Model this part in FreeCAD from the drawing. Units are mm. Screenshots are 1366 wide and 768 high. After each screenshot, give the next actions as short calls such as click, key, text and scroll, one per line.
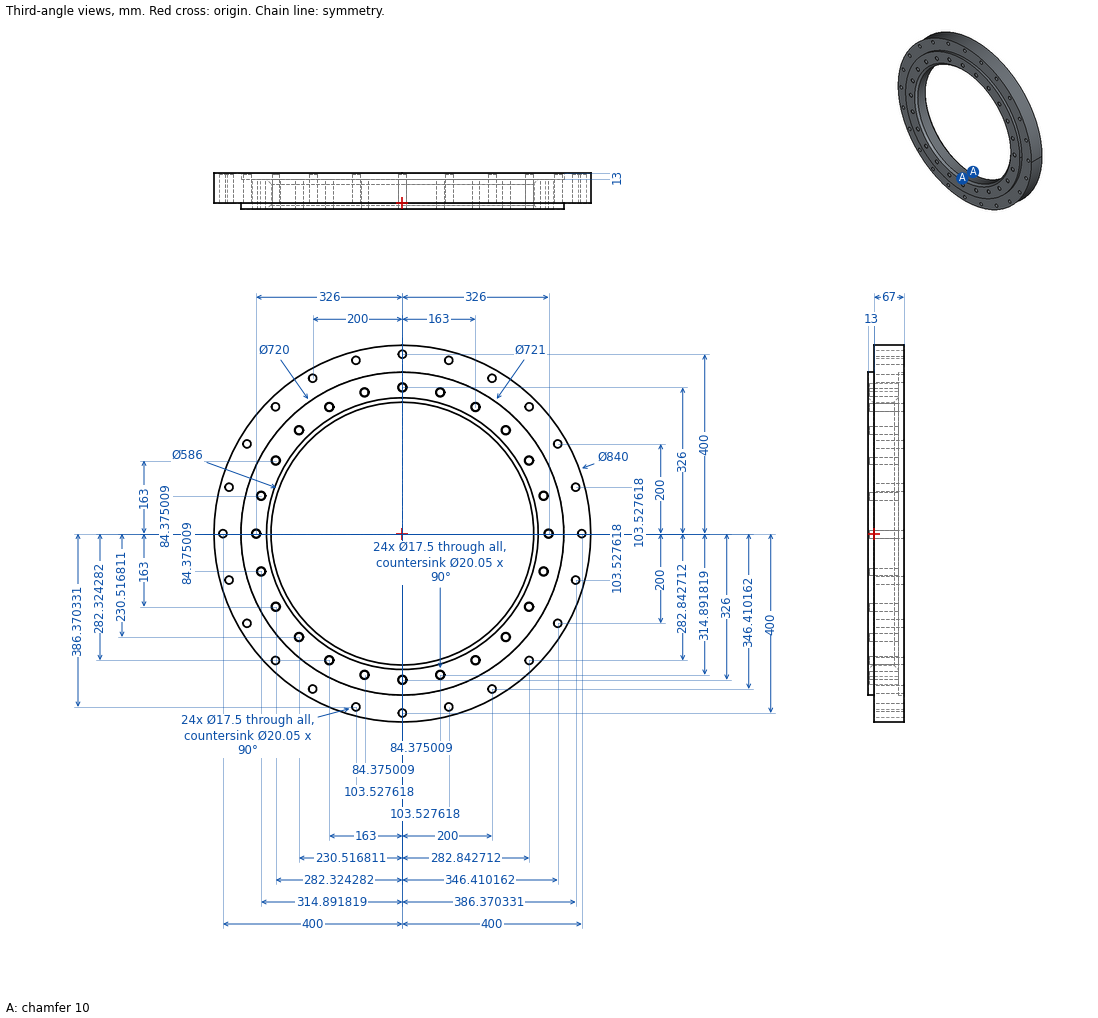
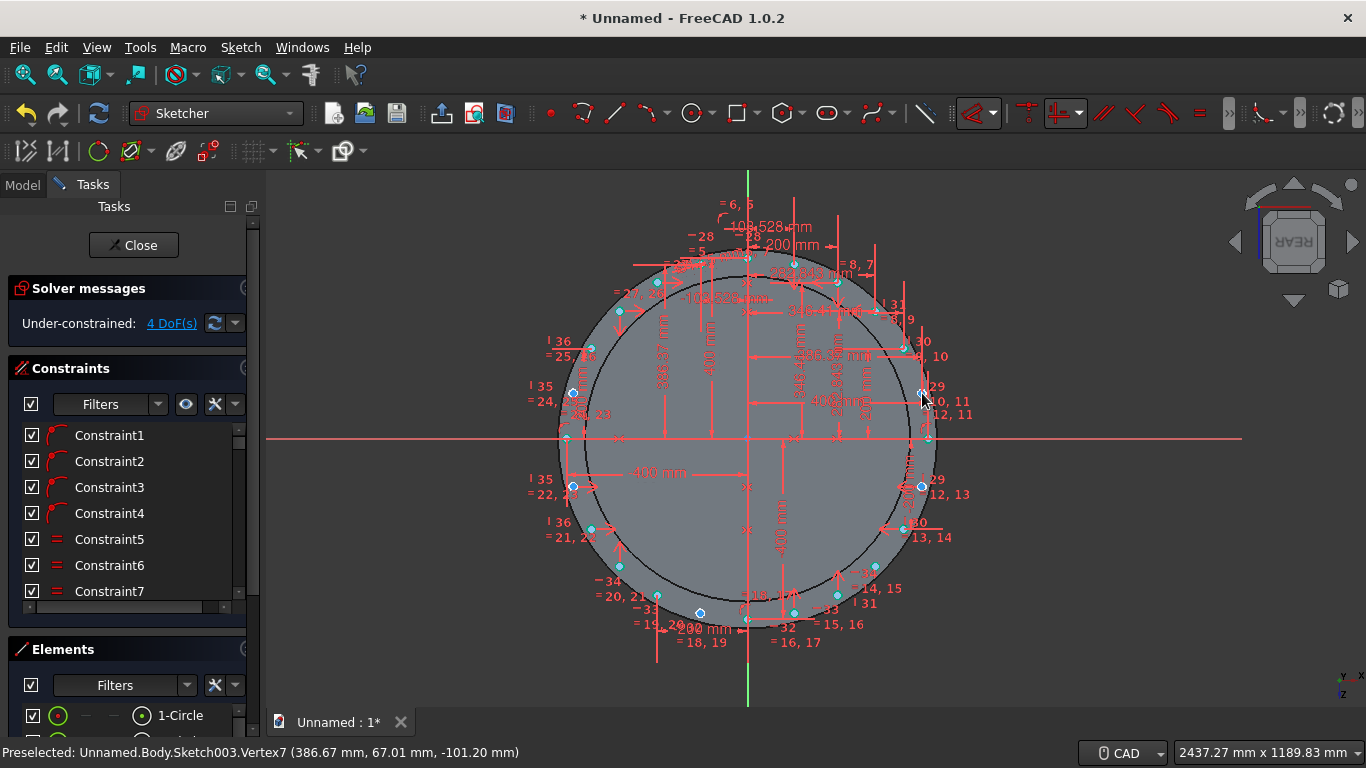
click(922, 393)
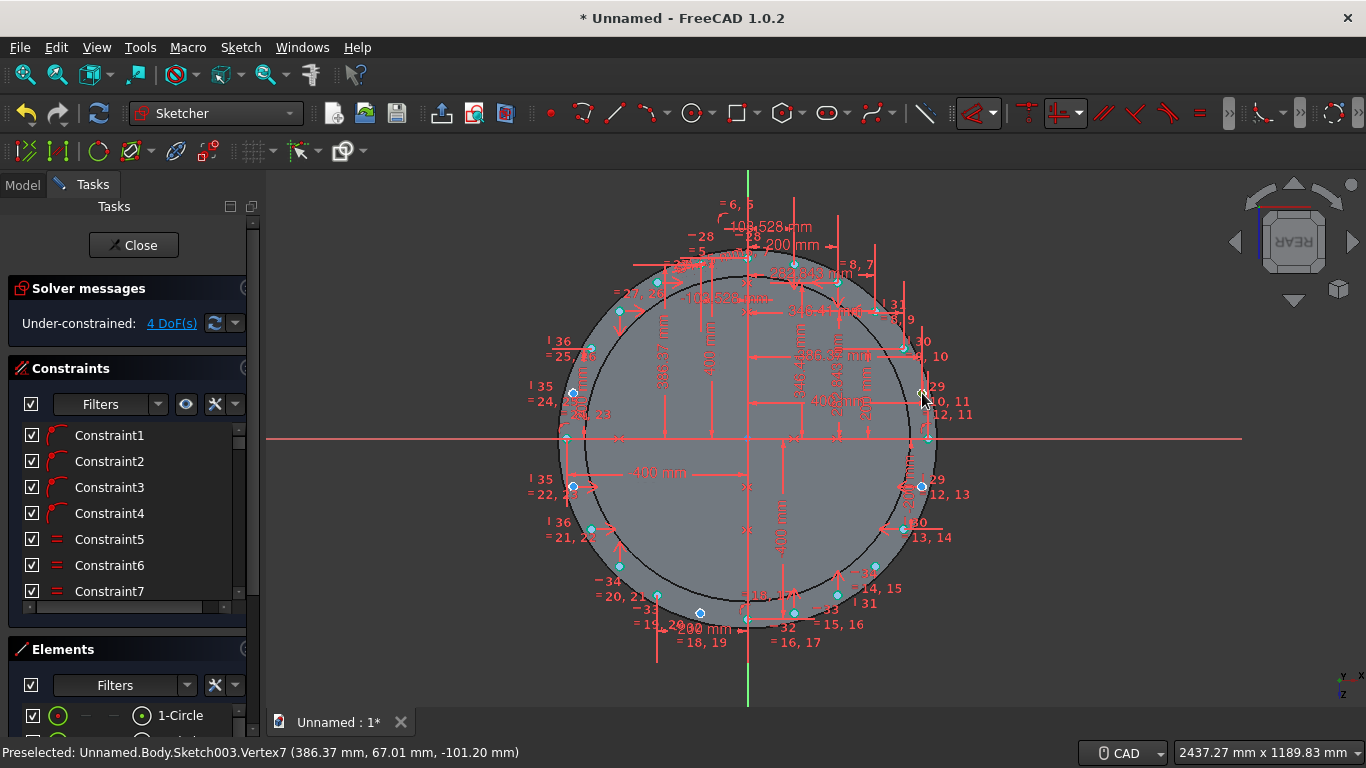
click(996, 114)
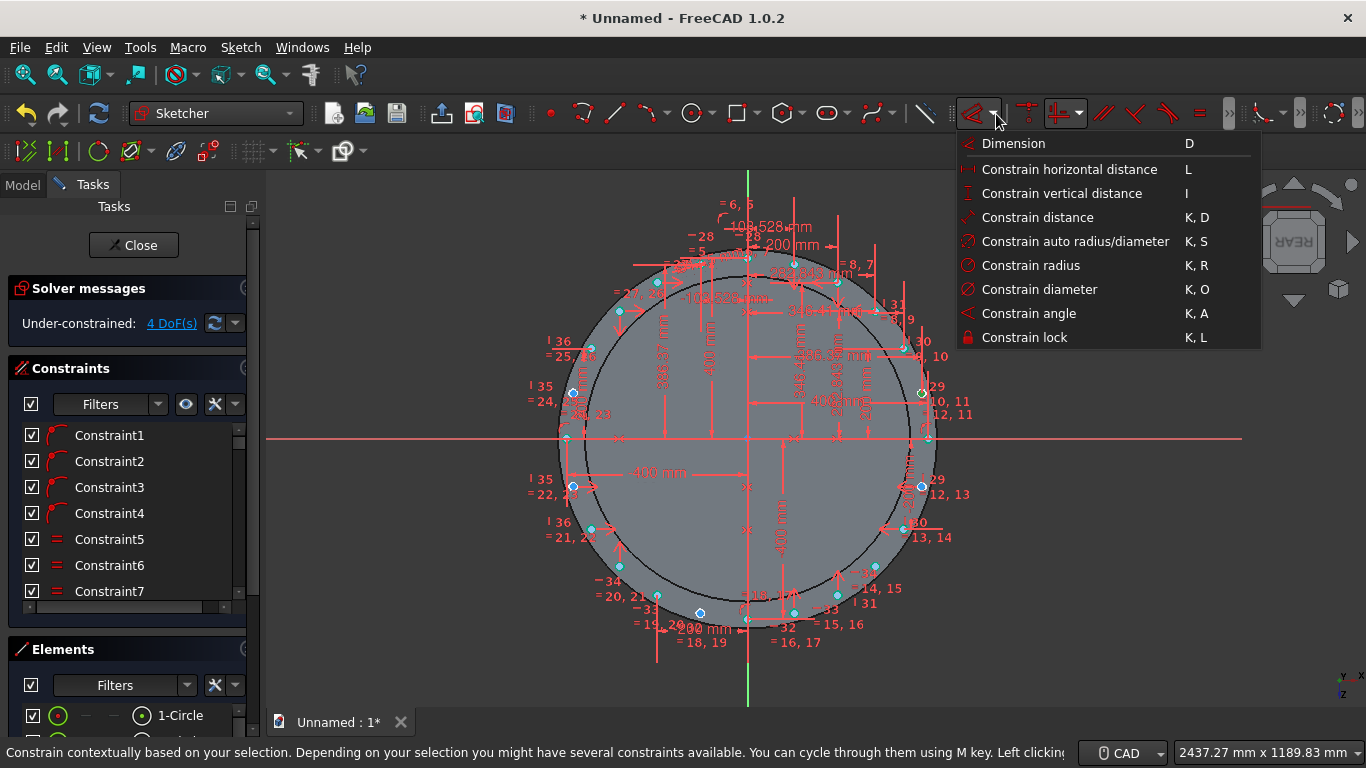
click(1109, 193)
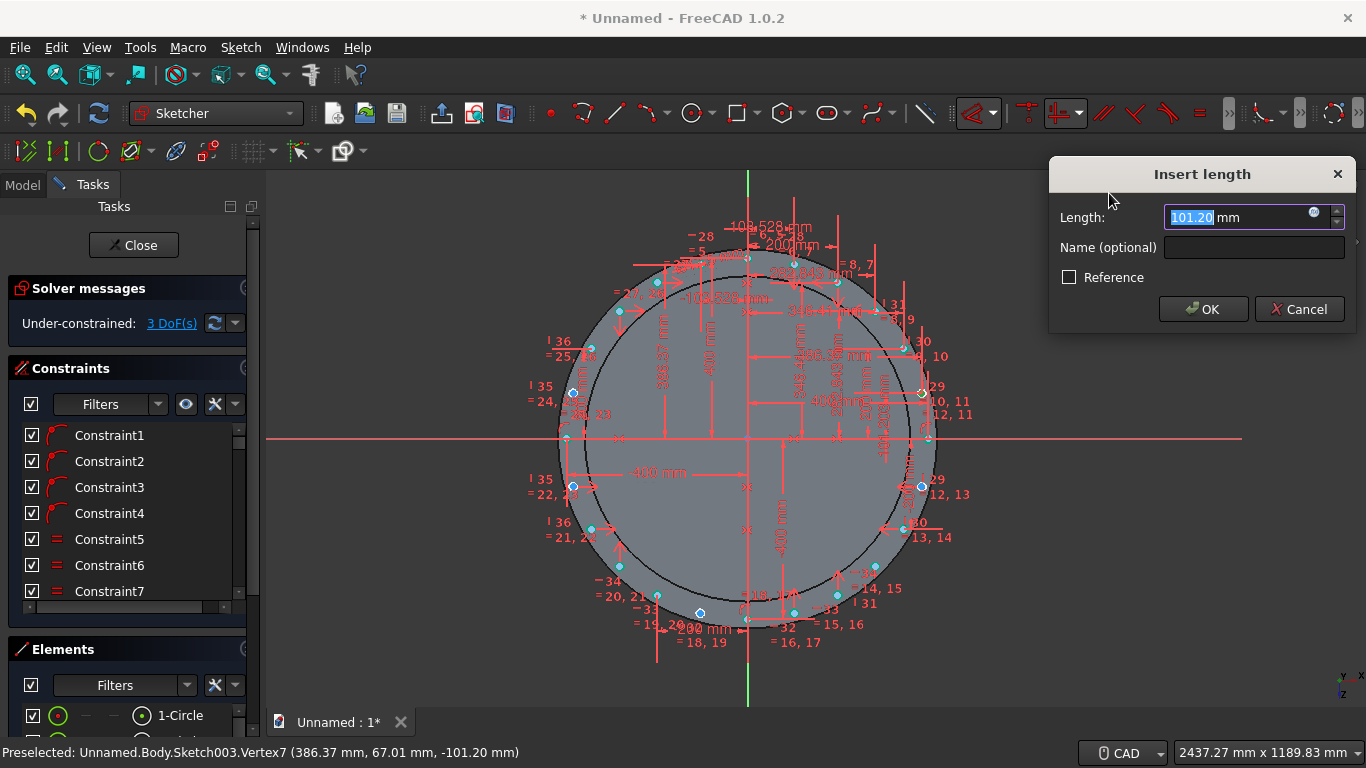
text(103.527618)
key(Return)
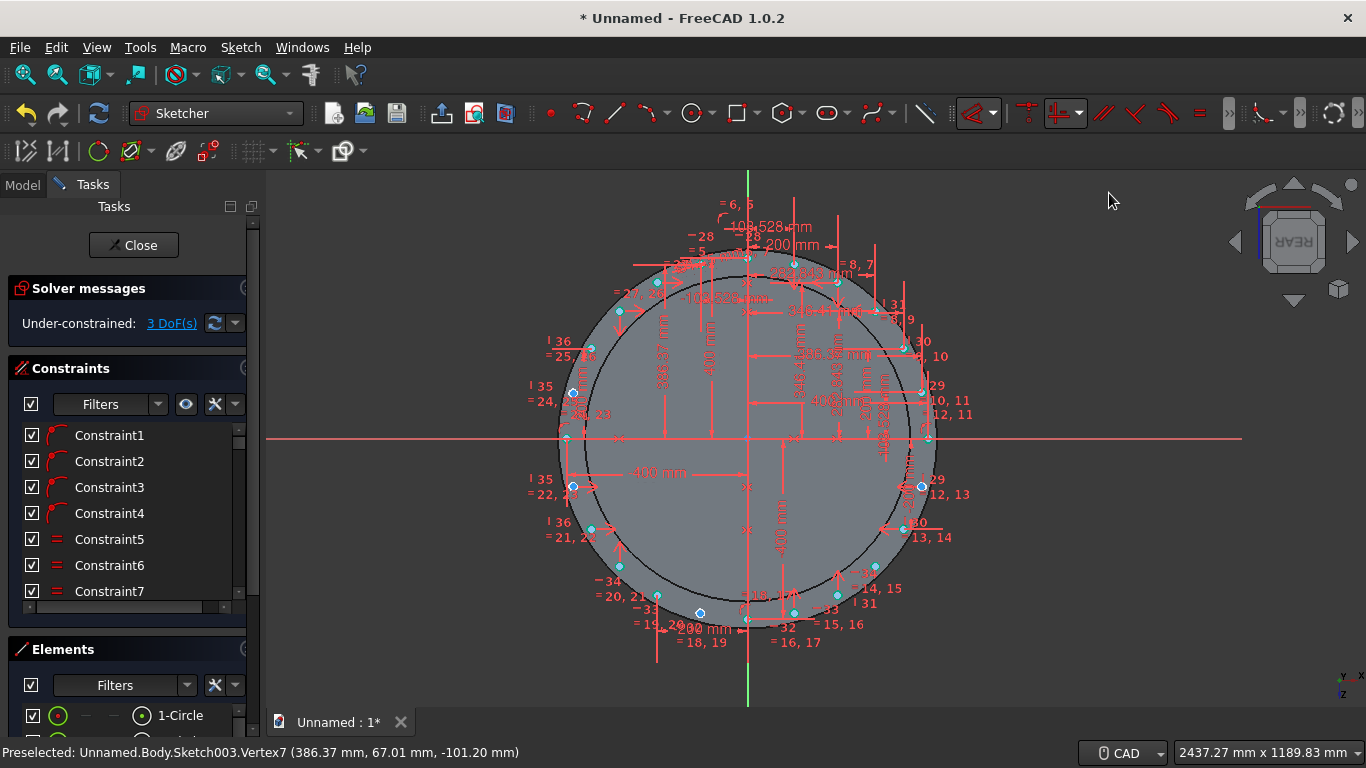
scroll(922, 487, up, 4)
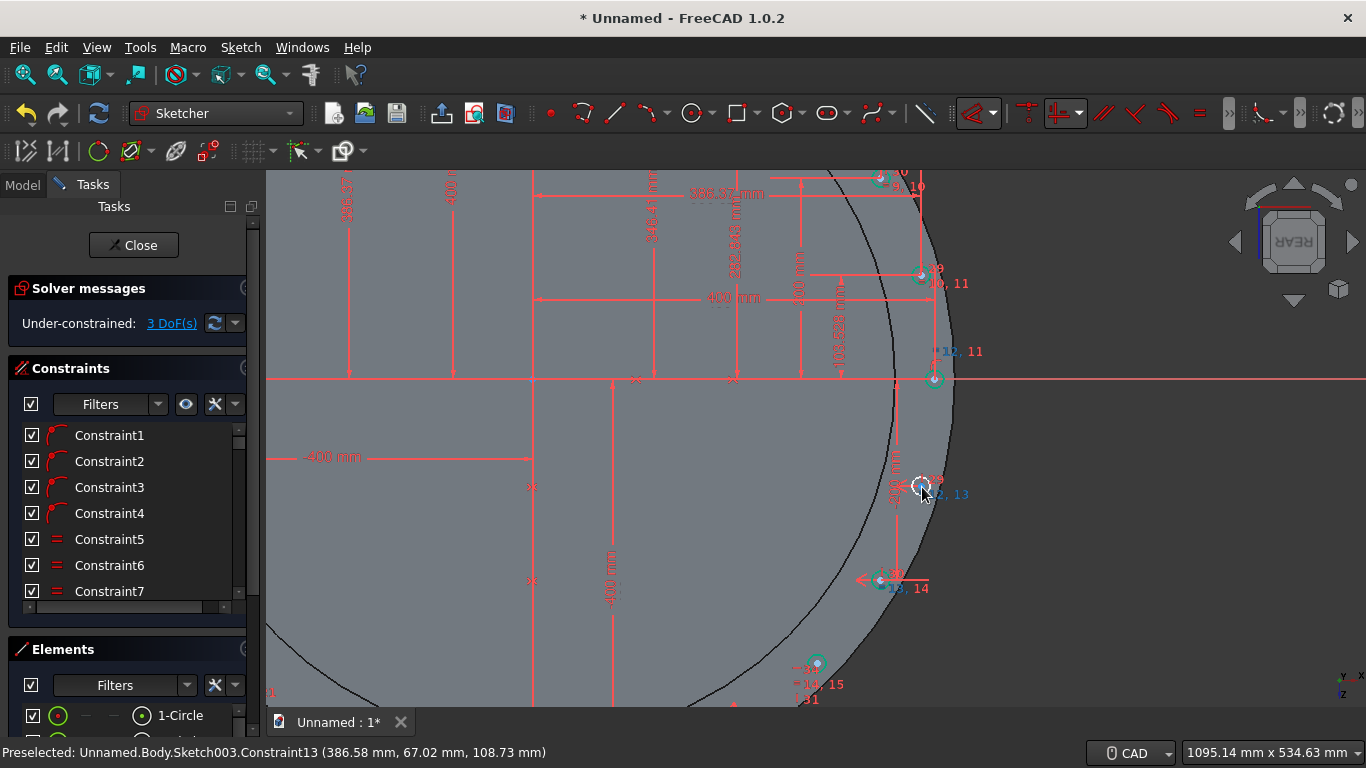
scroll(921, 486, up, 4)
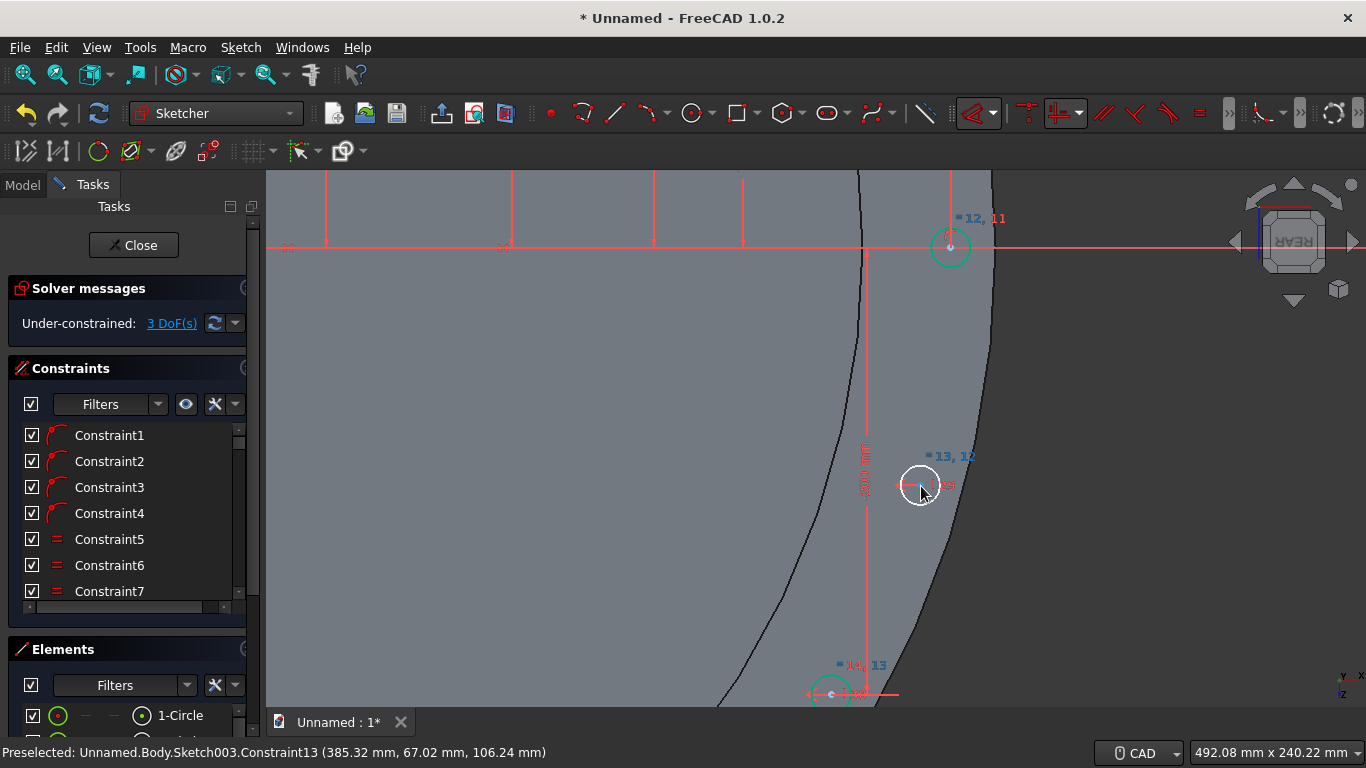
click(920, 485)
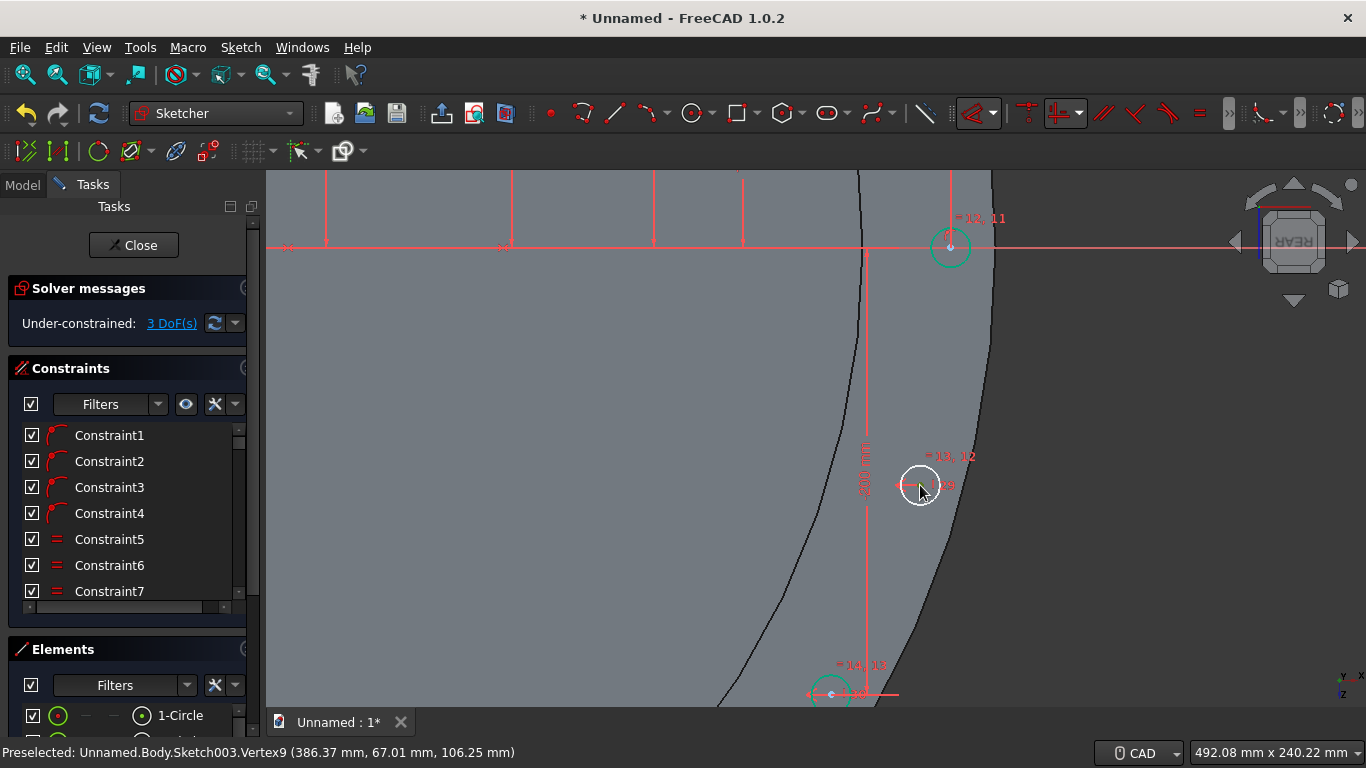
key(i)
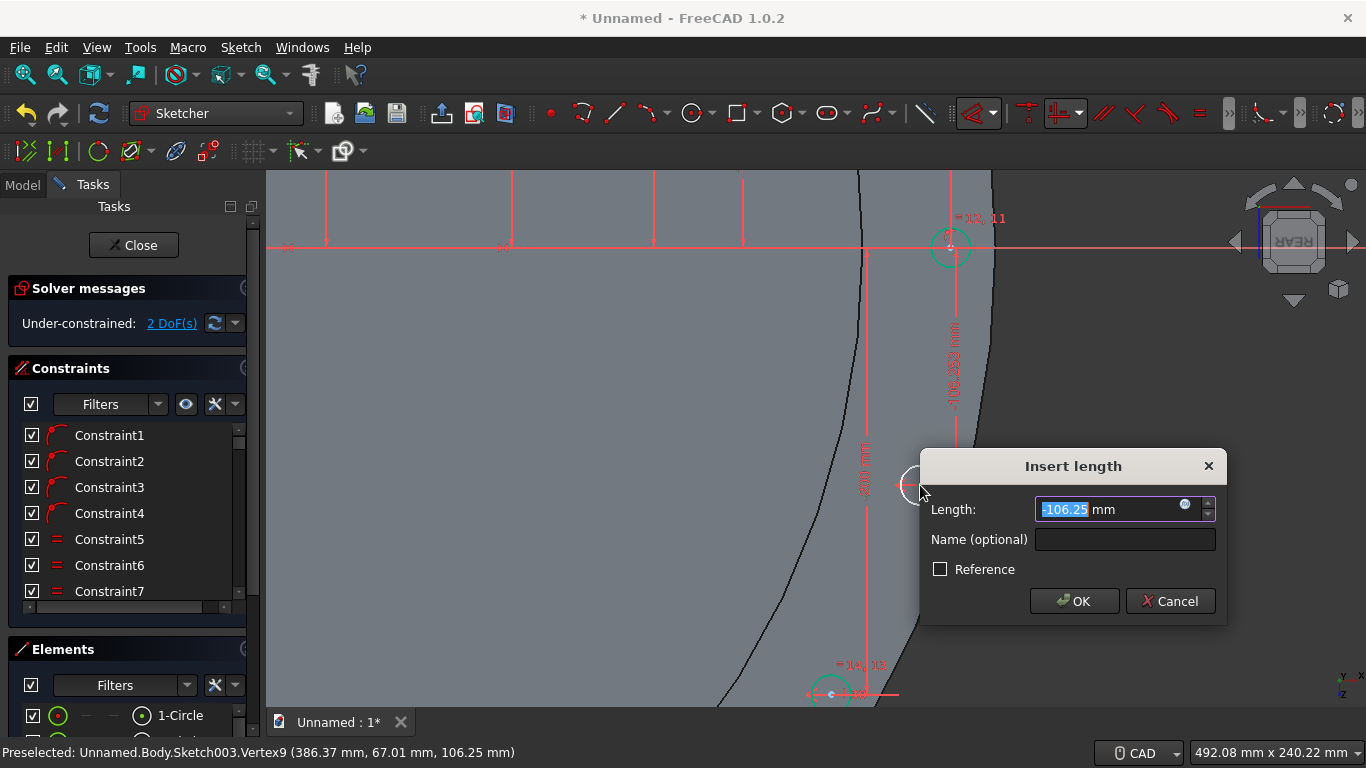
text(-103.527618)
key(Return)